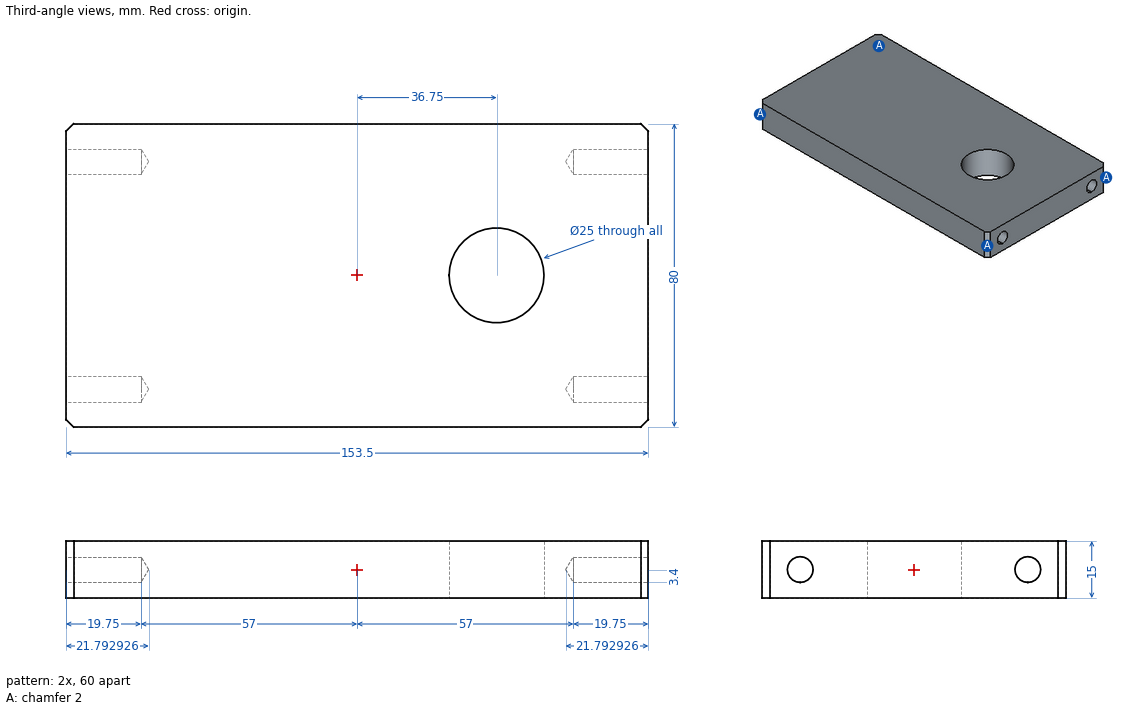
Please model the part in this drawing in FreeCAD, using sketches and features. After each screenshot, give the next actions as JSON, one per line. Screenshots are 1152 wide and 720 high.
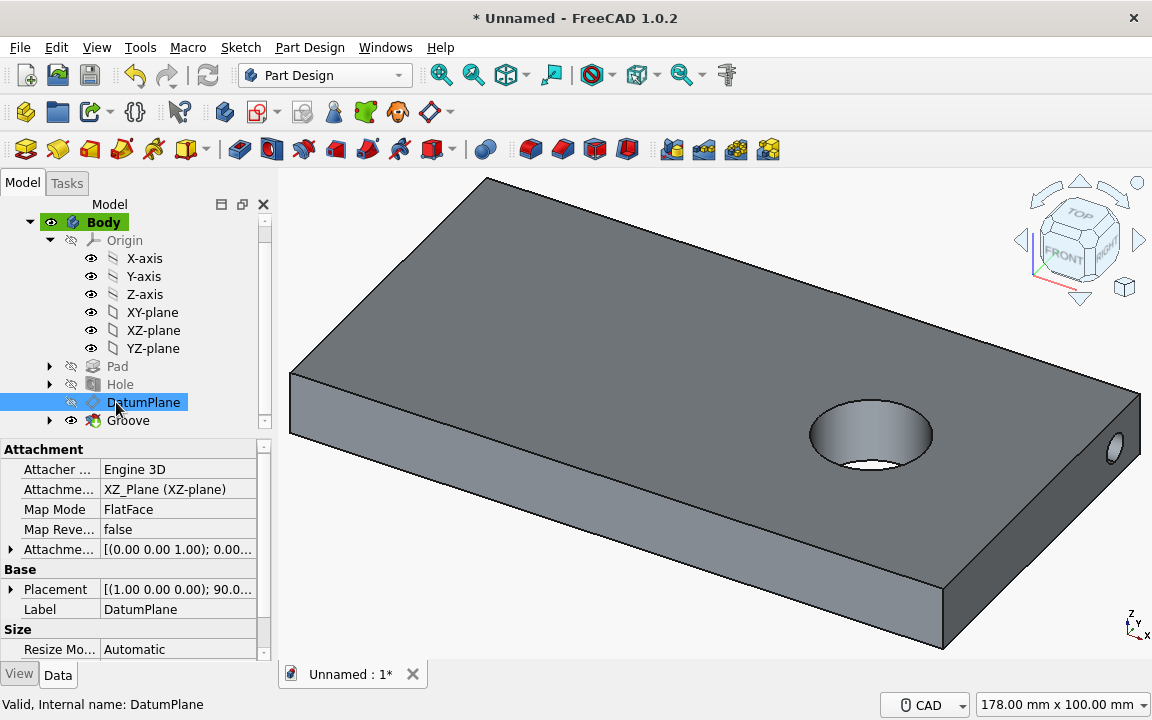
{"action": "left_click", "coordinate": [116, 420]}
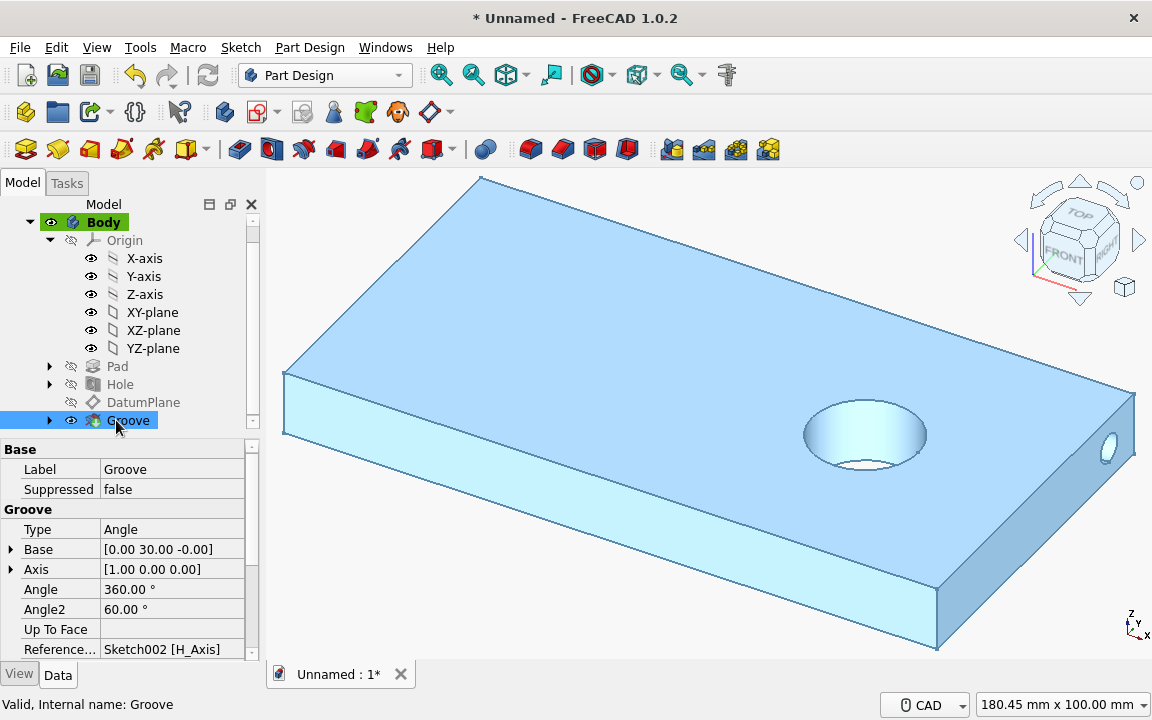
{"action": "left_click", "coordinate": [704, 150]}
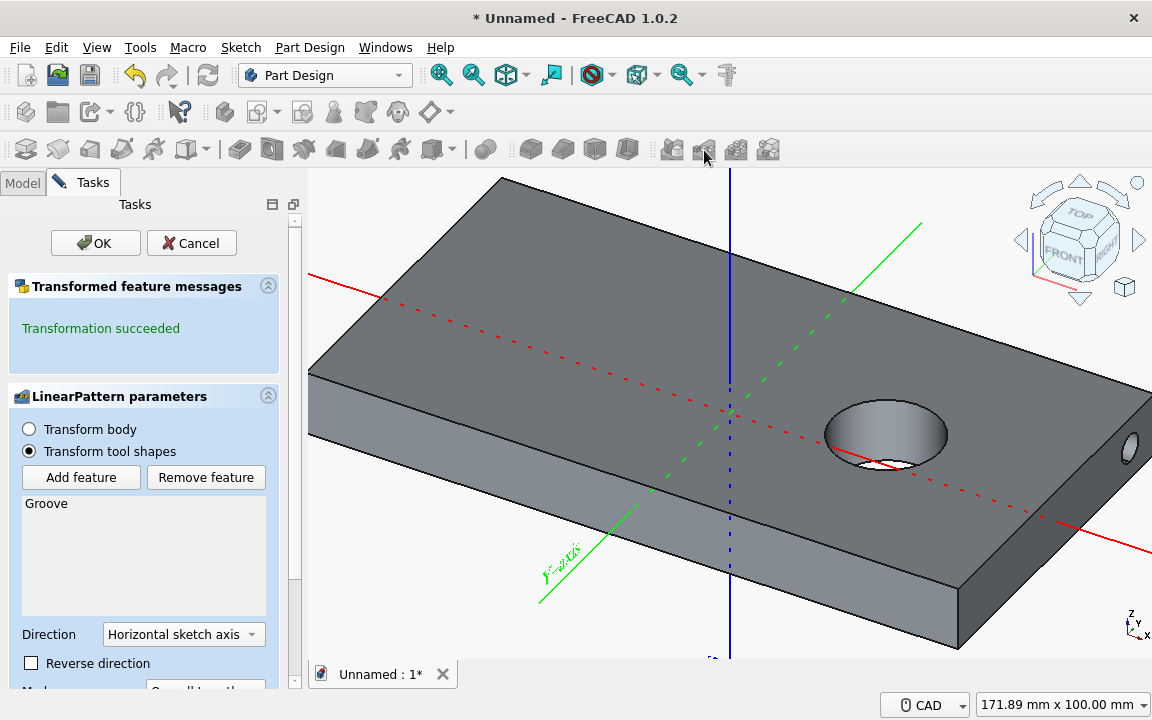
{"action": "left_click", "coordinate": [184, 634]}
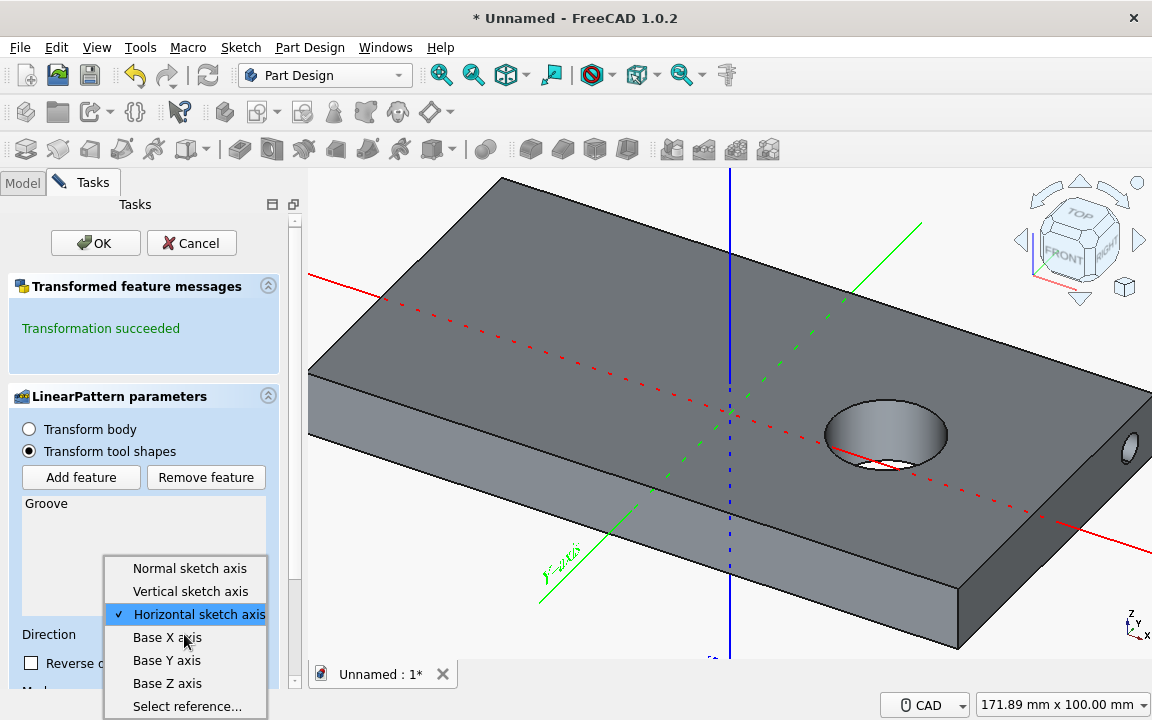
{"action": "left_click", "coordinate": [184, 660]}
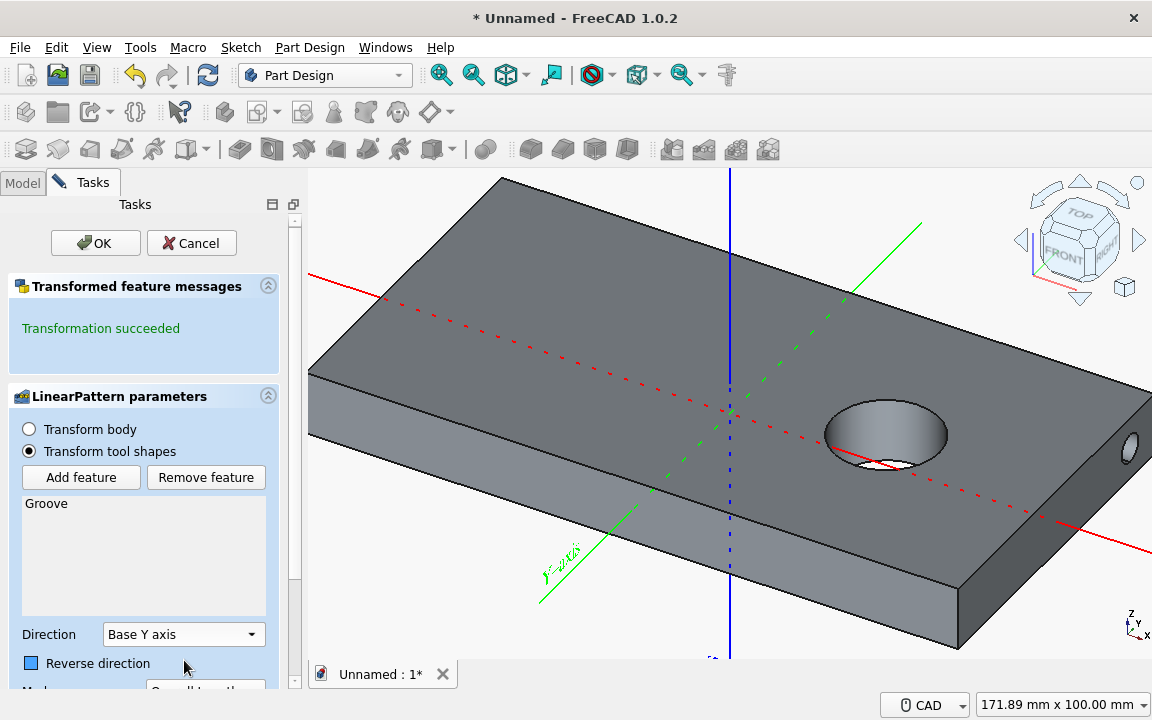
{"action": "scroll", "coordinate": [295, 451], "scroll_direction": "down", "scroll_amount": 2}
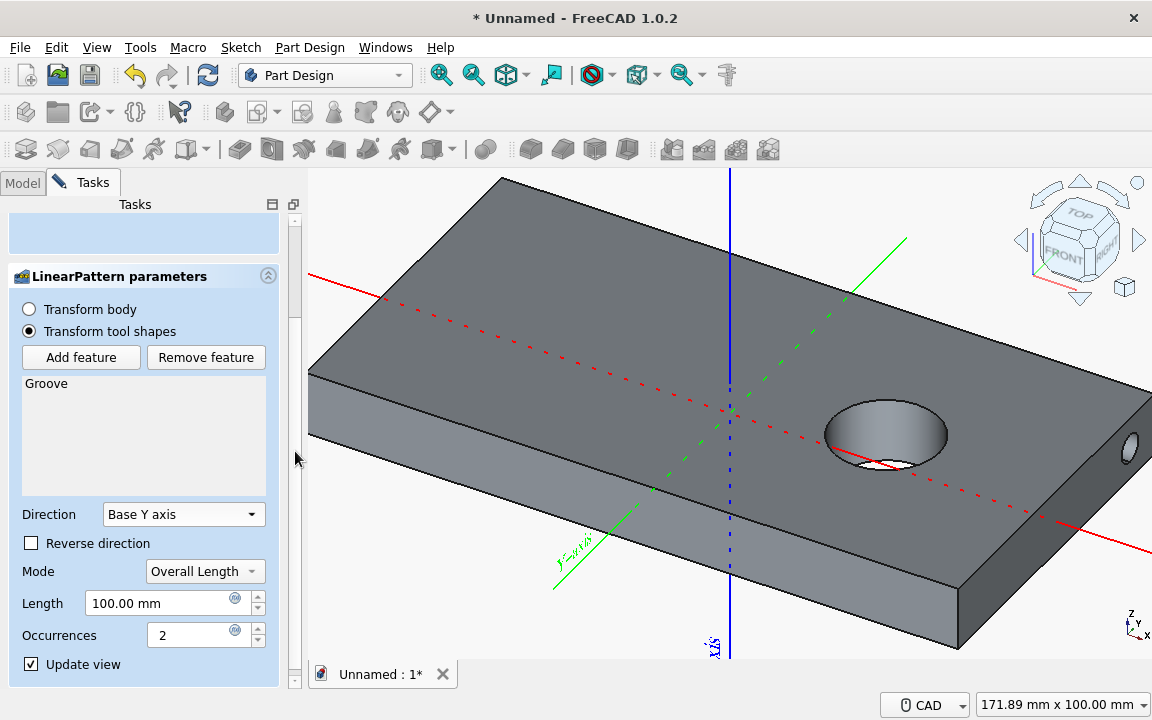
{"action": "left_click", "coordinate": [206, 572]}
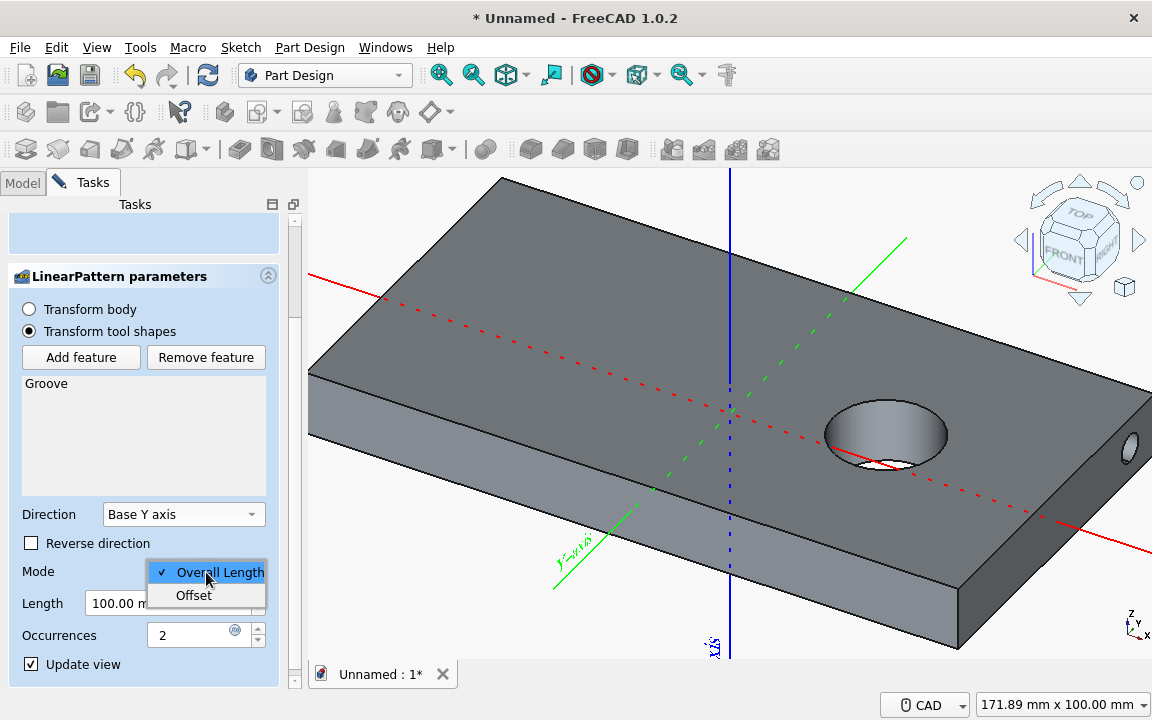
{"action": "left_click", "coordinate": [206, 596]}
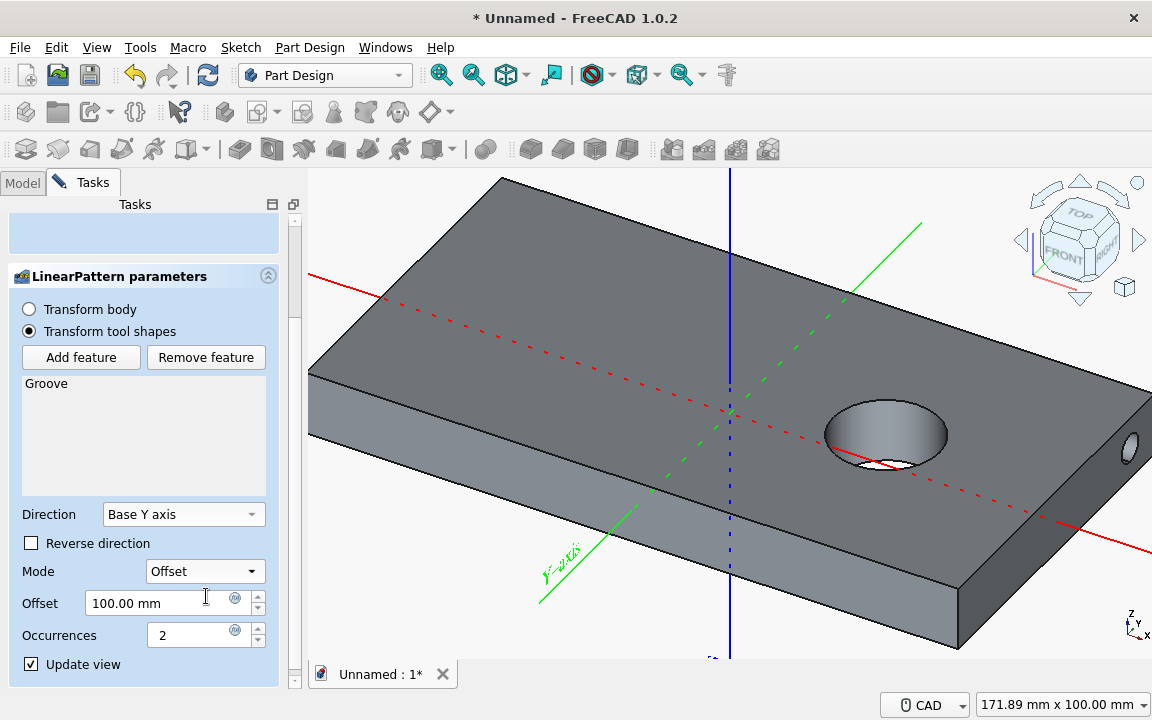
{"action": "triple_click", "coordinate": [168, 603]}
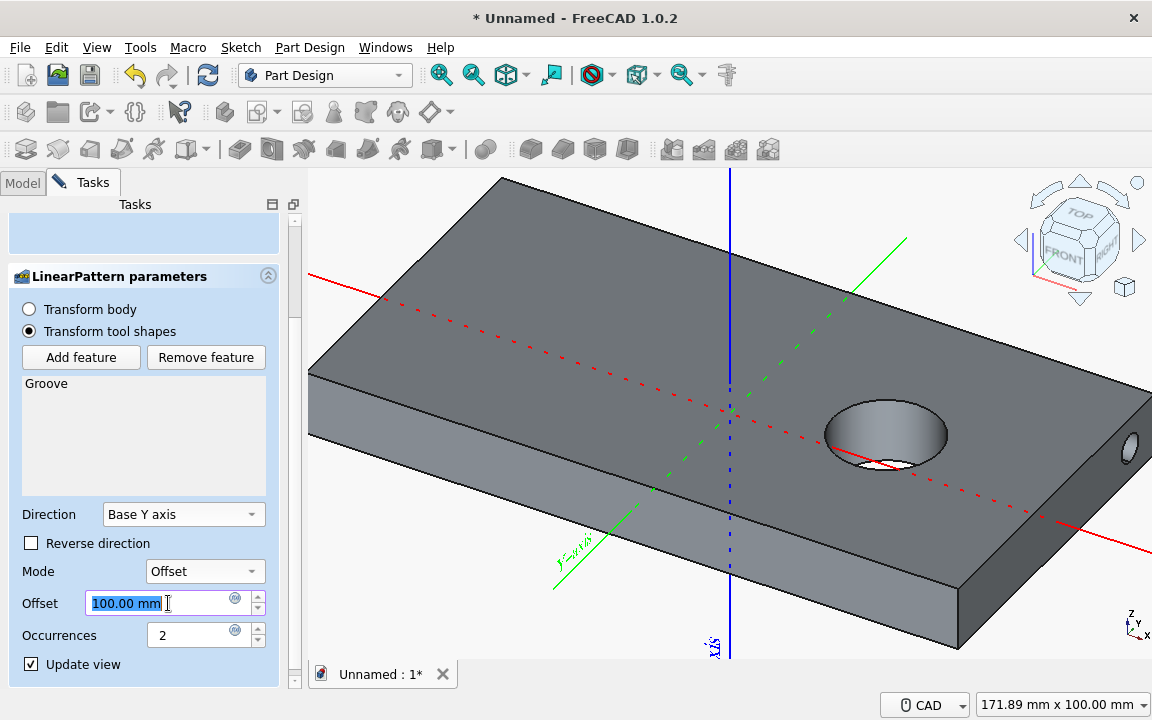
{"action": "type", "text": "60"}
{"action": "key", "text": "Tab"}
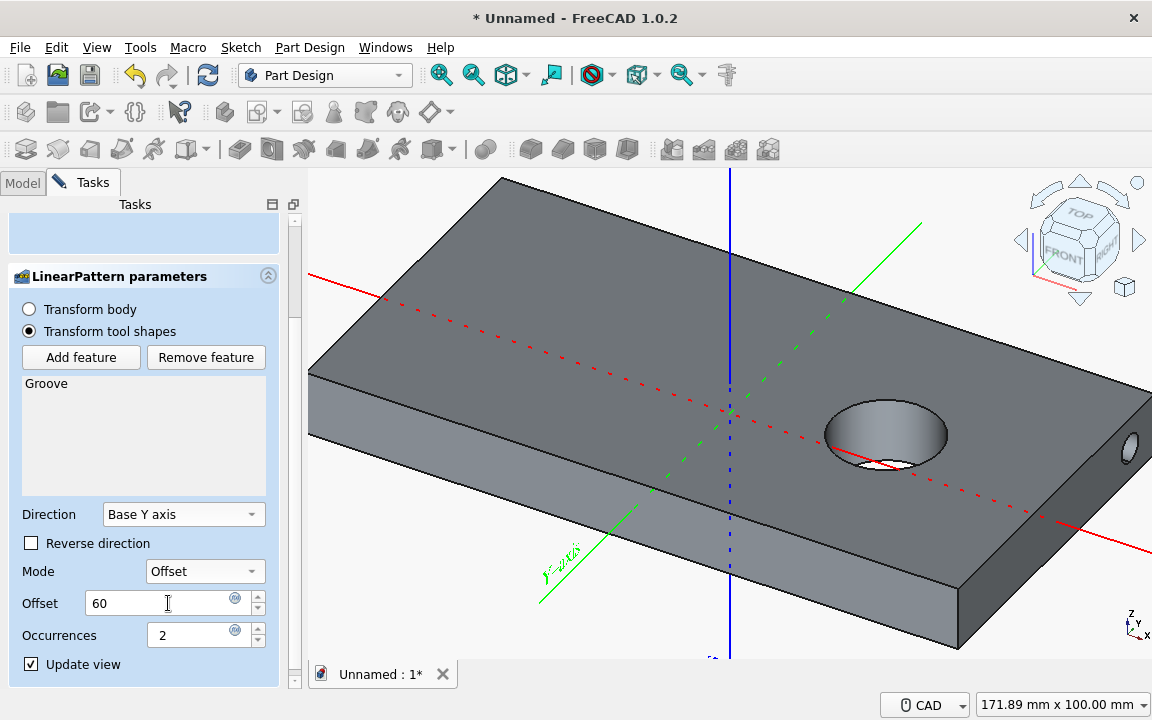
{"action": "triple_click", "coordinate": [198, 635]}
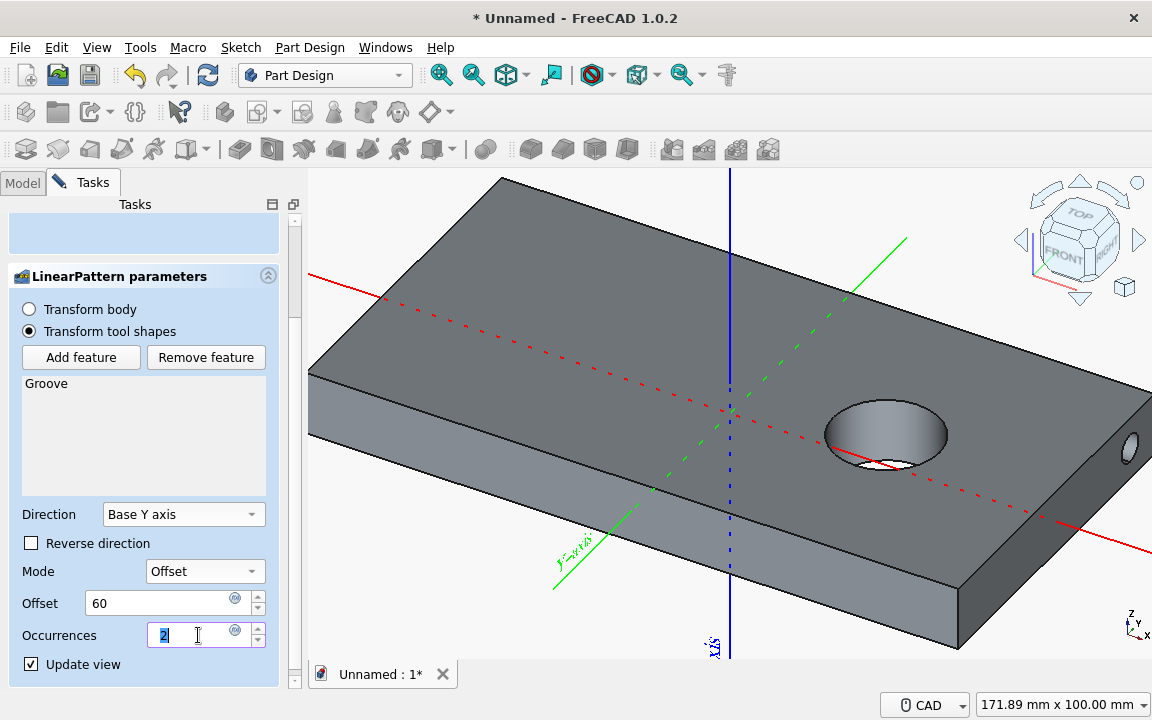
{"action": "type", "text": "2"}
{"action": "key", "text": "Tab"}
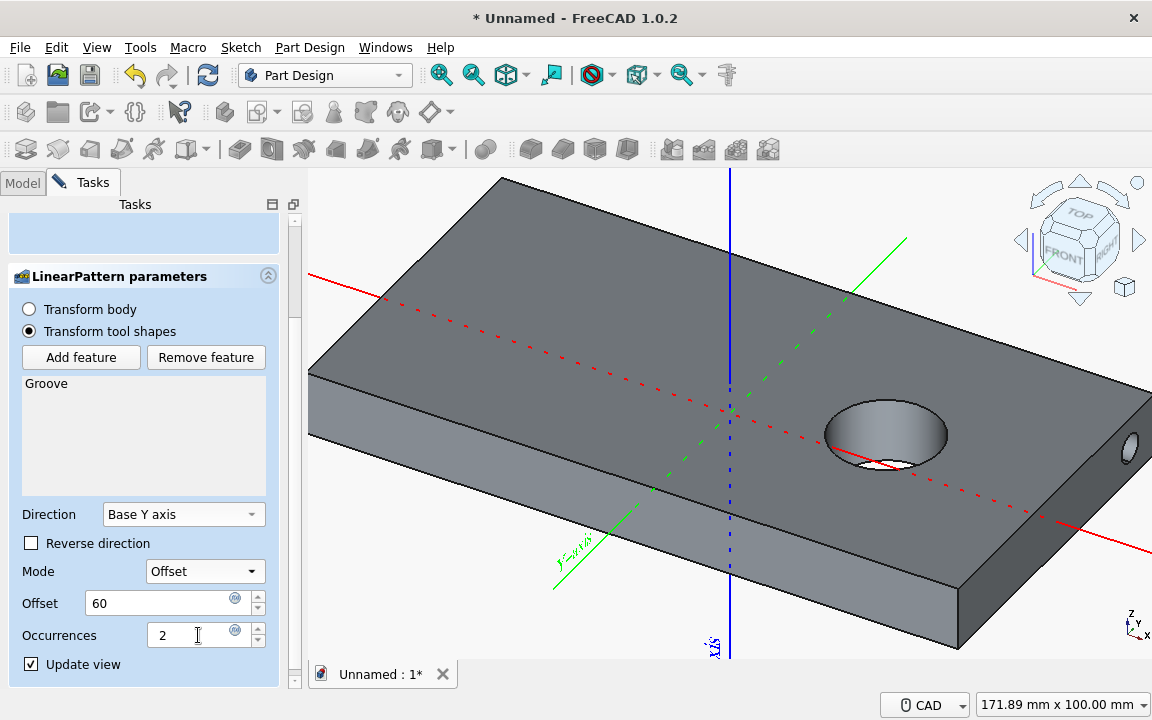
{"action": "left_click", "coordinate": [30, 543]}